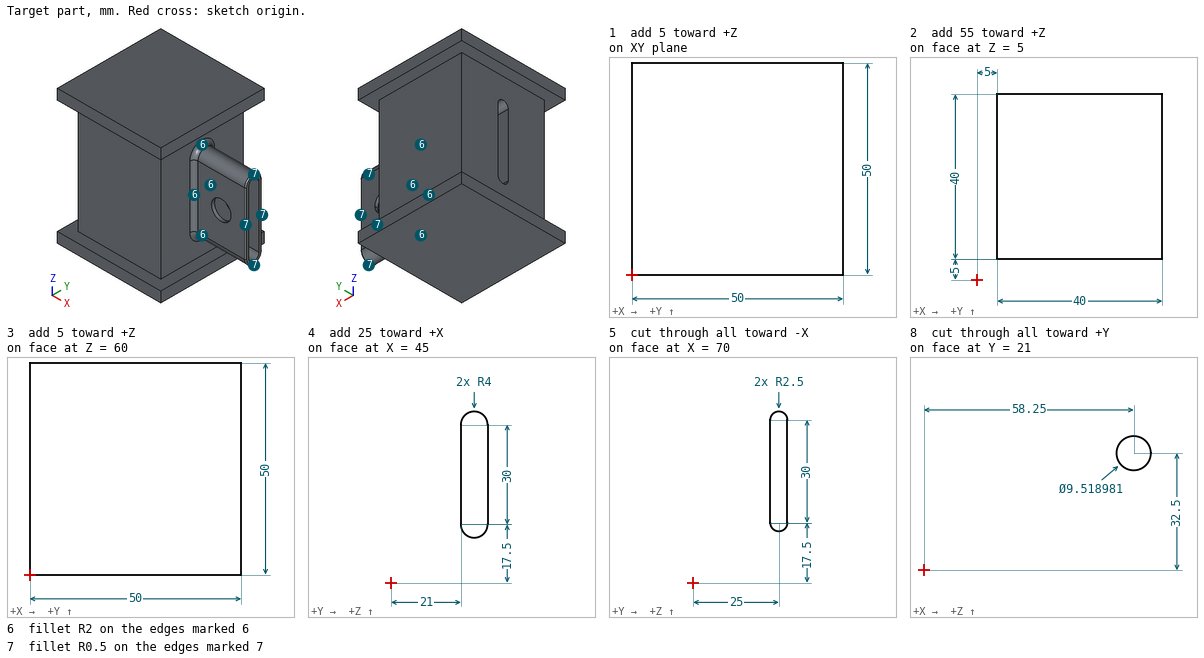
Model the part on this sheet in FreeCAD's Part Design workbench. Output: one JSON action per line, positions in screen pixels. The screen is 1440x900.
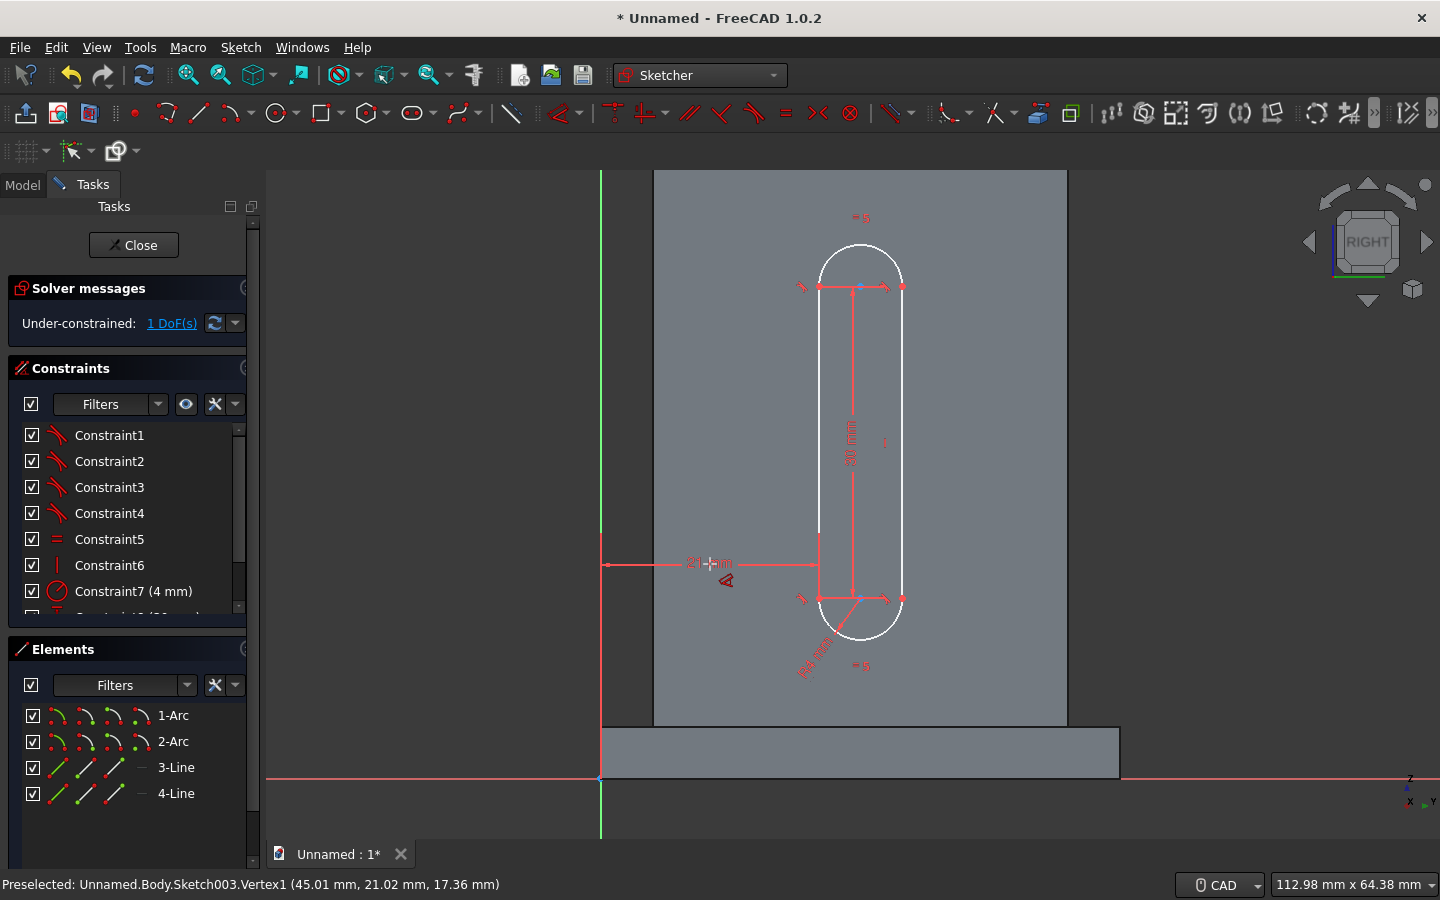
{"action": "left_click", "coordinate": [819, 598]}
{"action": "left_click", "coordinate": [567, 688]}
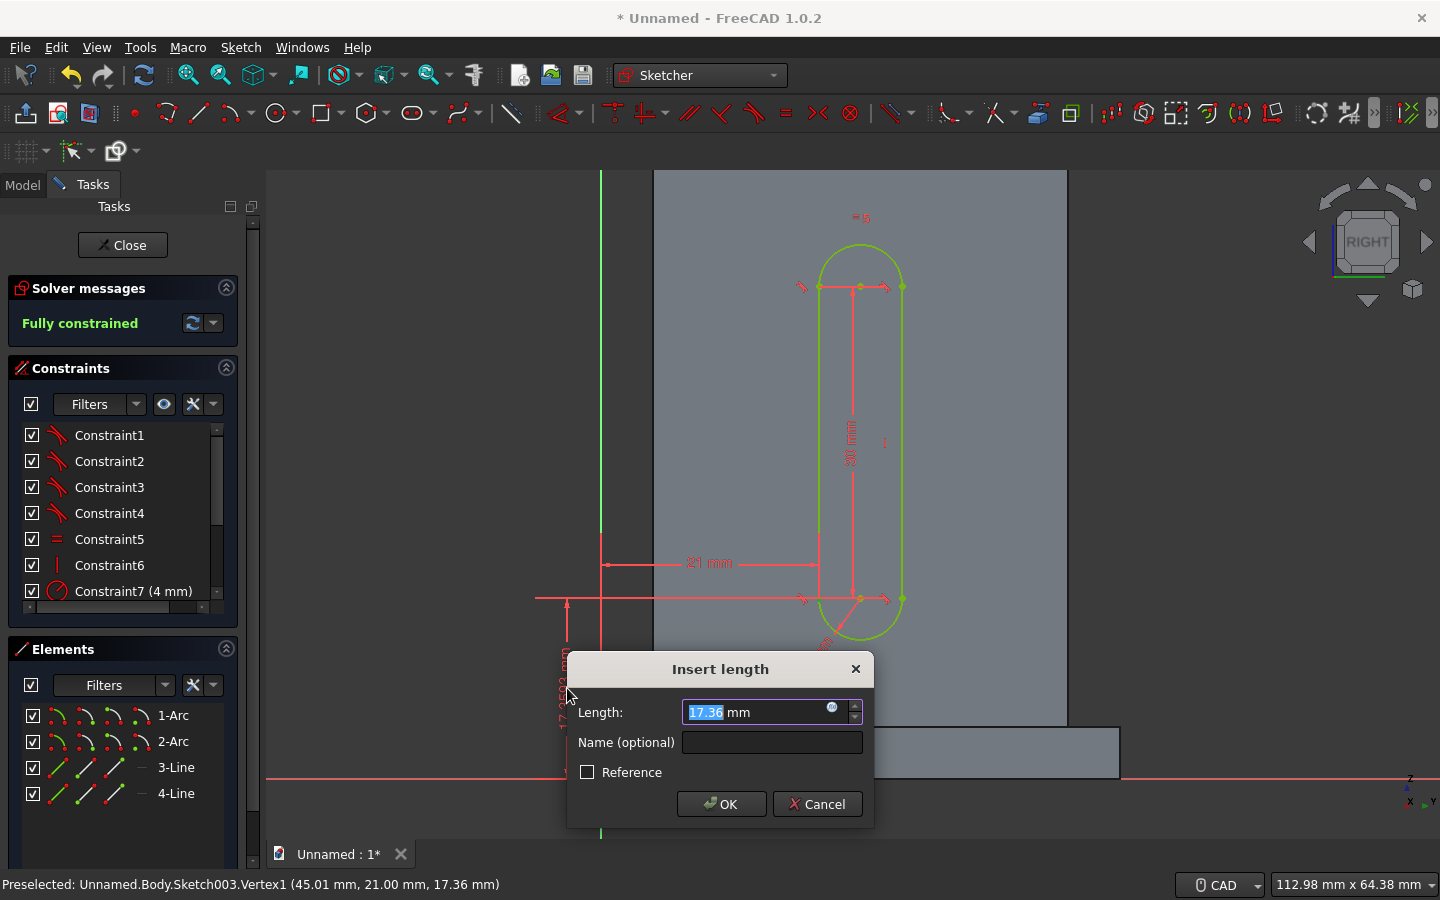
{"action": "type", "text": "17.5"}
{"action": "key", "text": "Return"}
{"action": "key", "text": "Escape"}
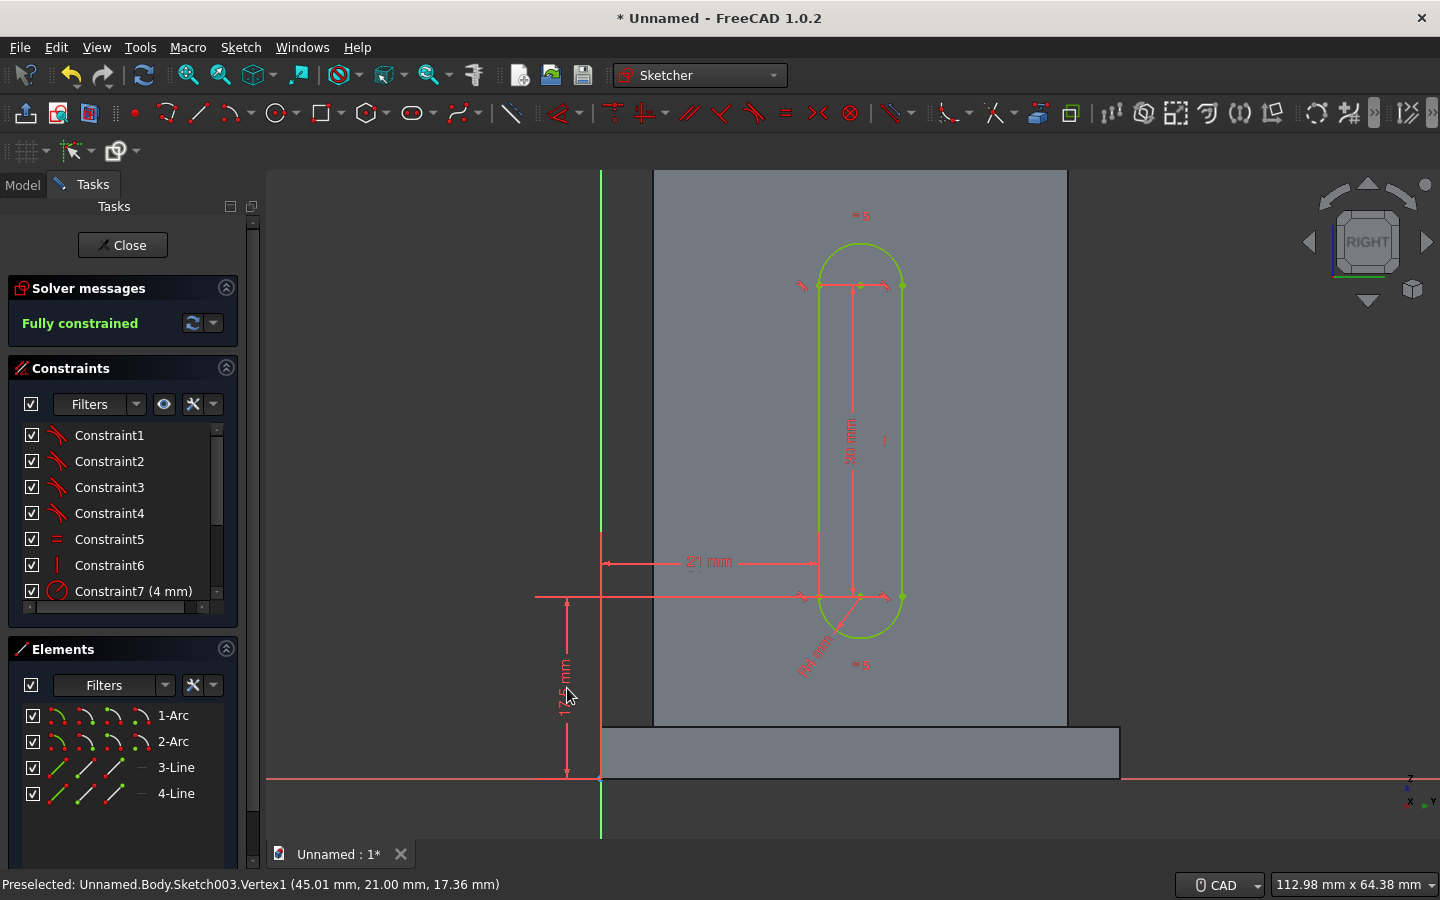
{"action": "left_click", "coordinate": [123, 245]}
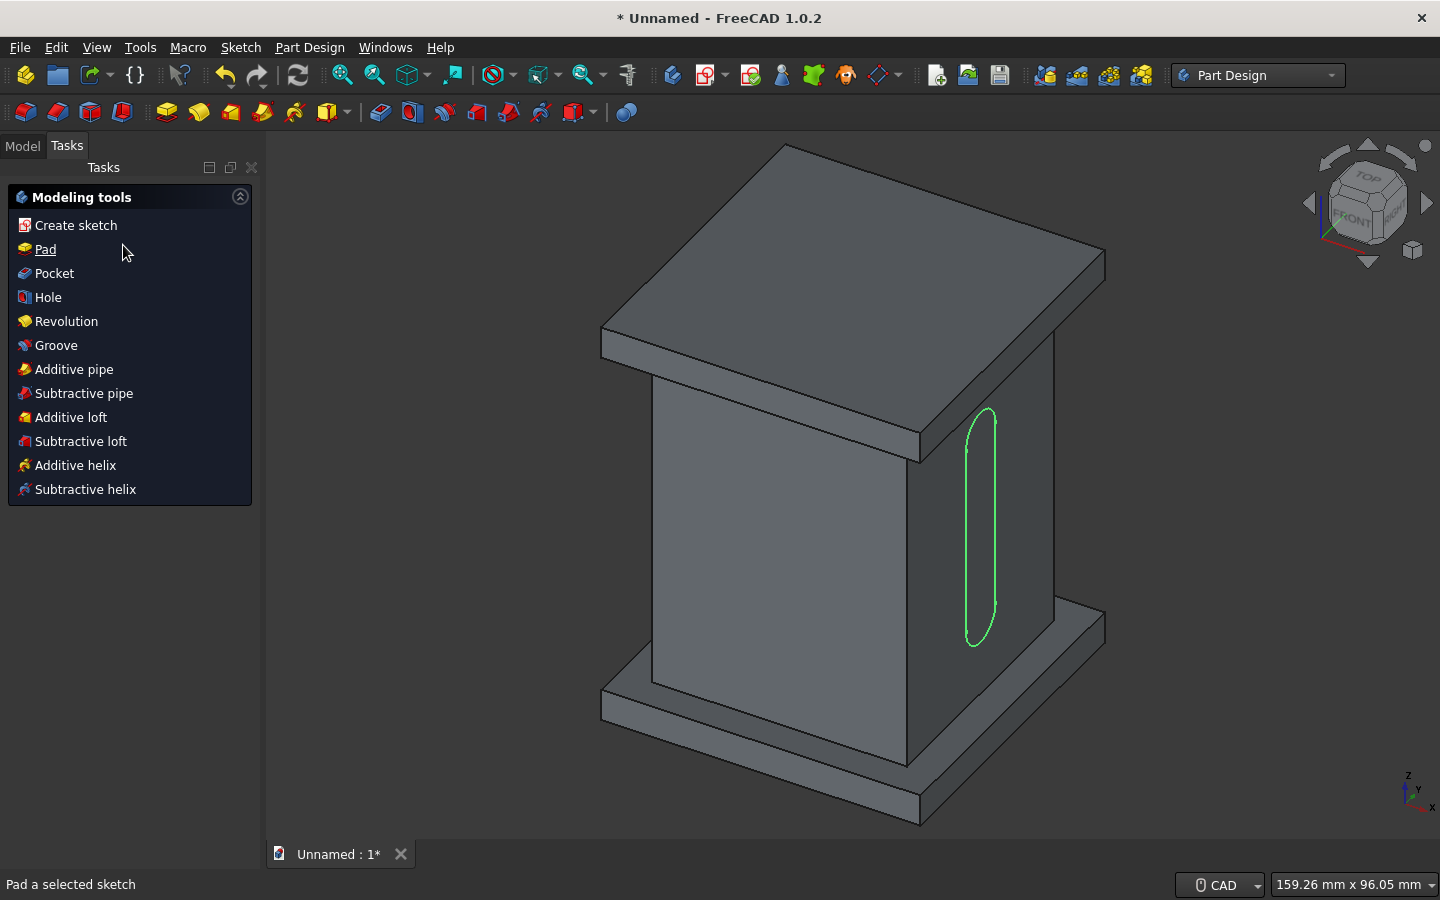
{"action": "left_click", "coordinate": [168, 112]}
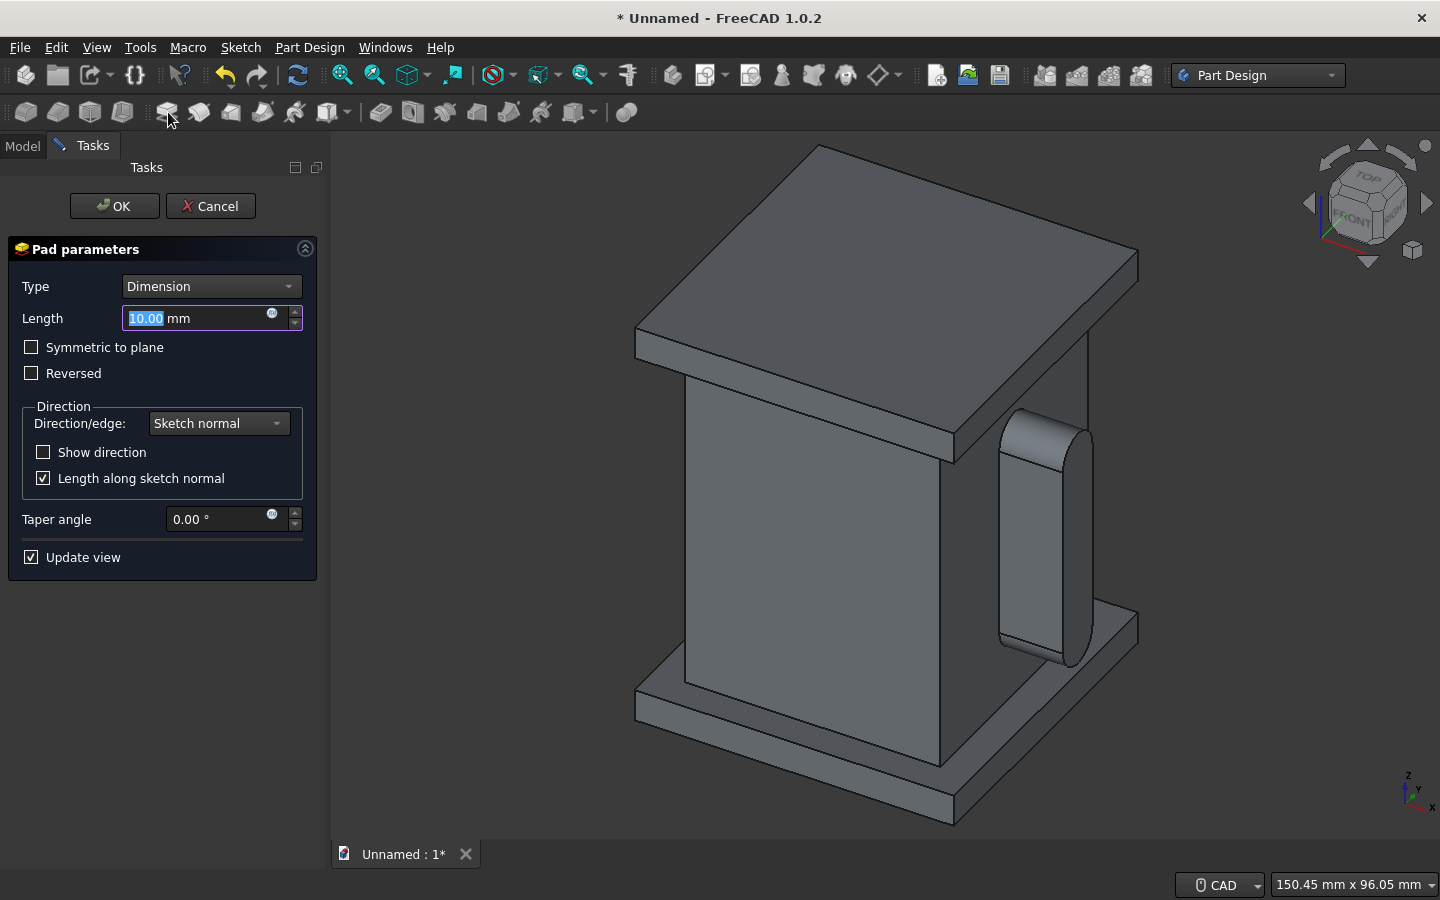
{"action": "type", "text": "25"}
{"action": "key", "text": "Tab"}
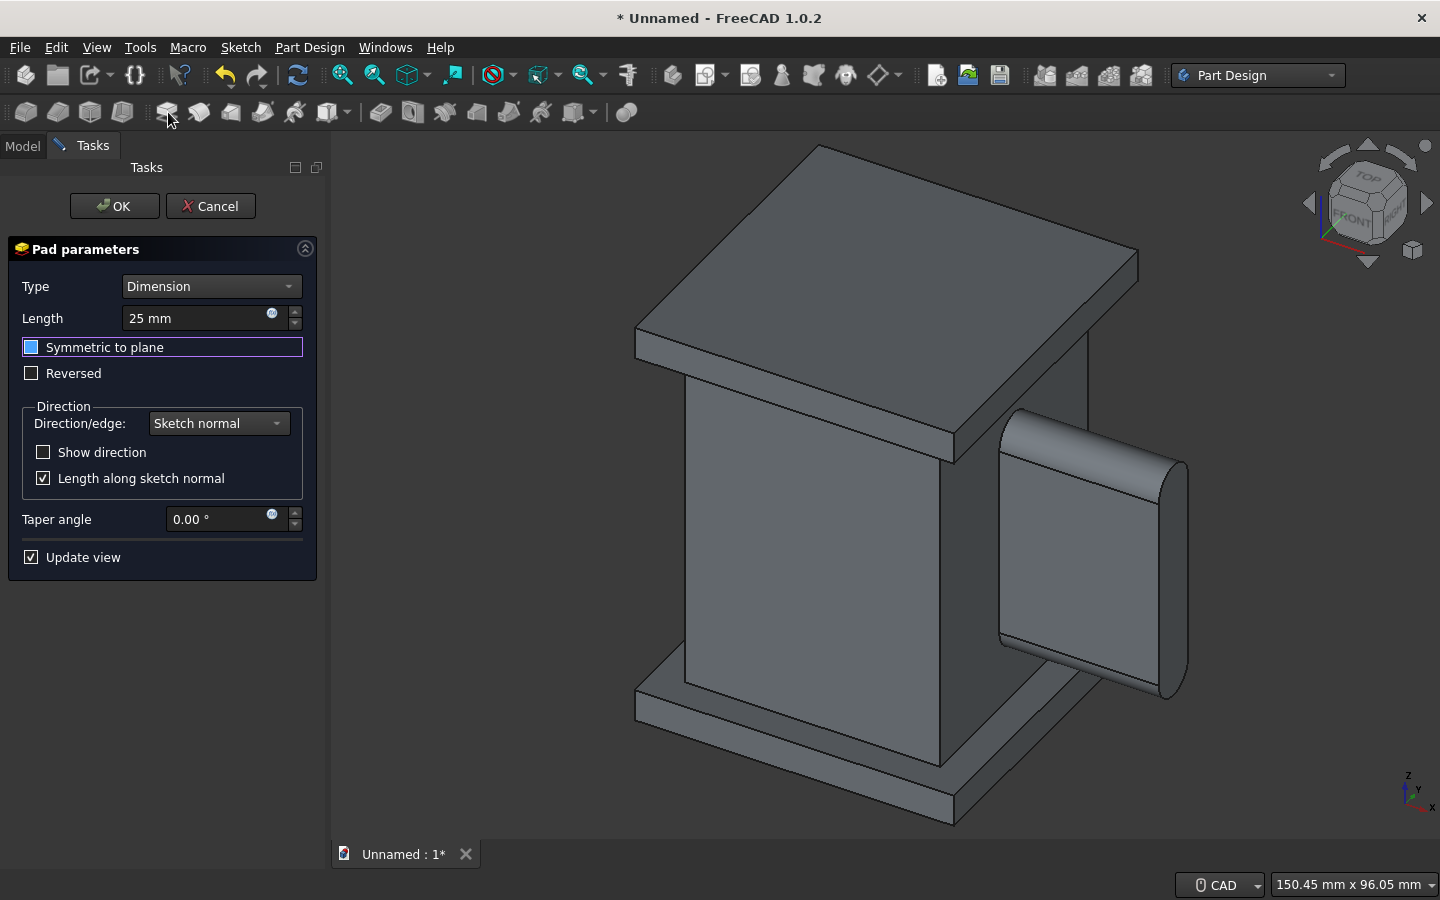
{"action": "left_click", "coordinate": [115, 206]}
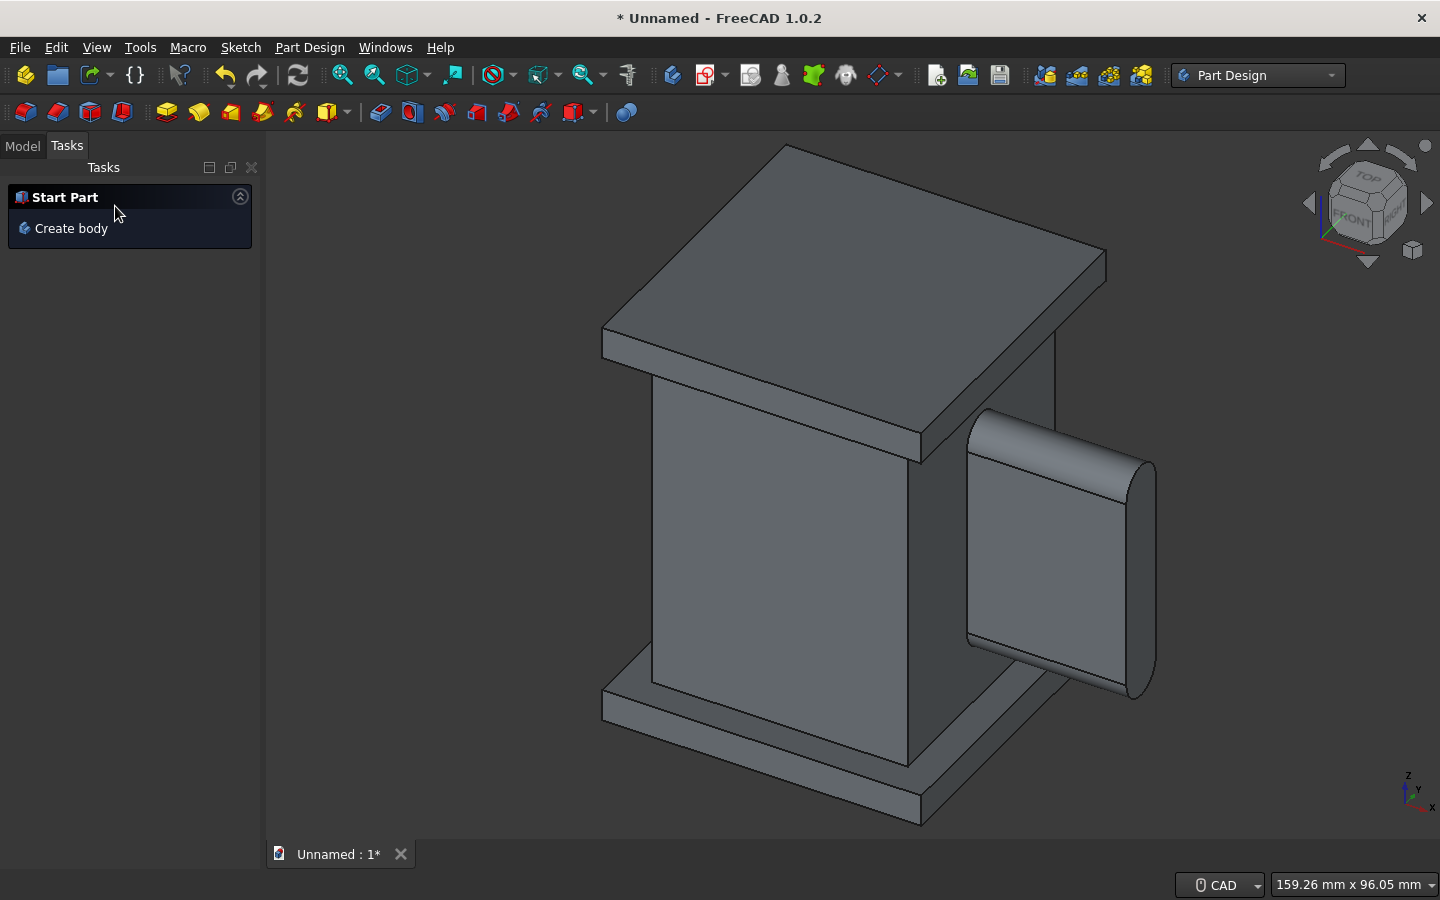
{"action": "left_click", "coordinate": [344, 76]}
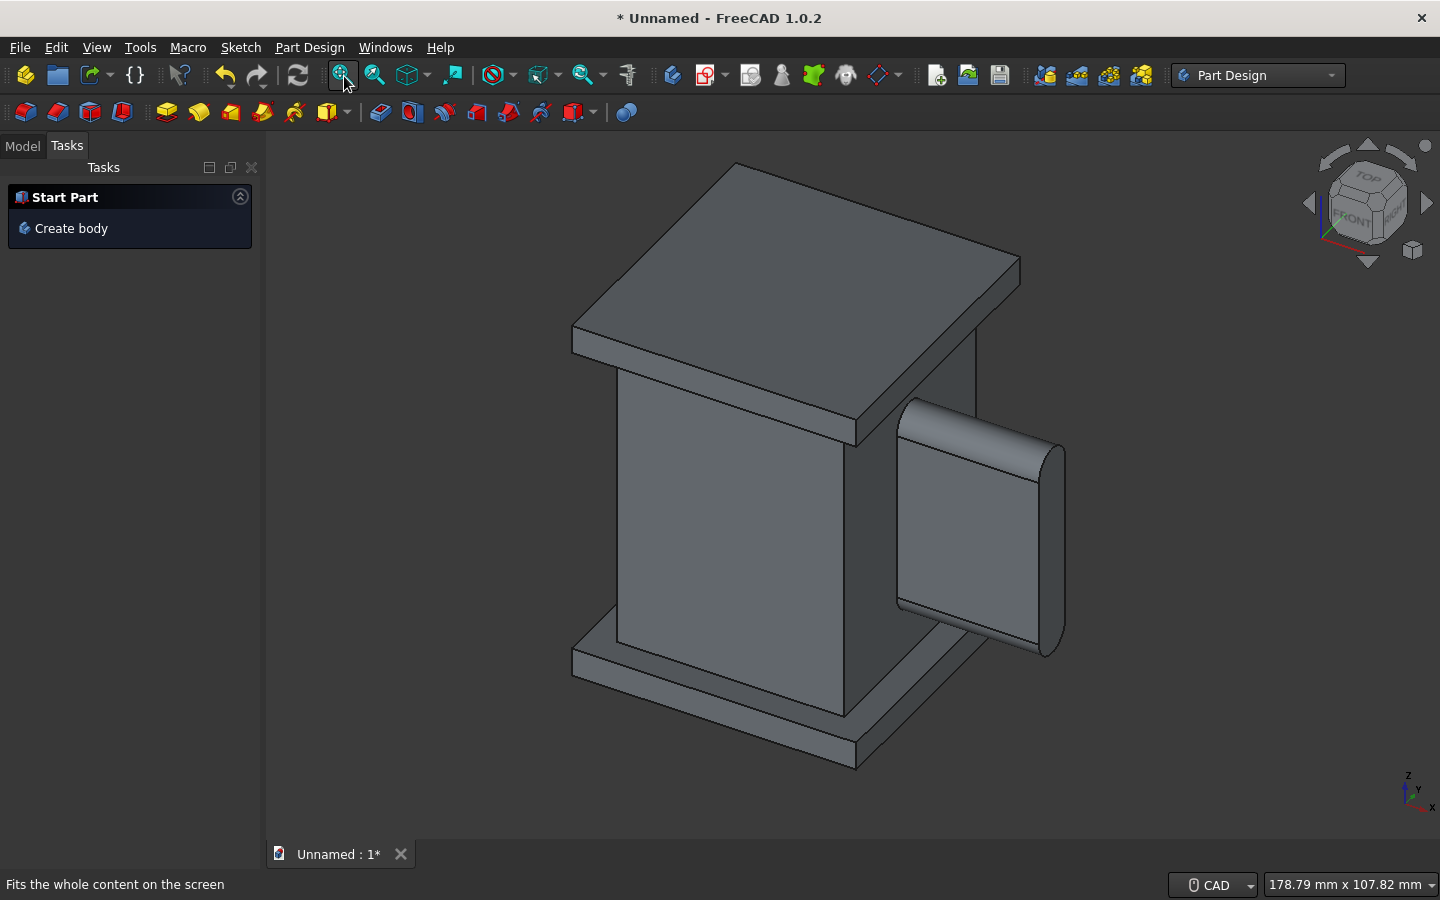
{"action": "left_click", "coordinate": [1052, 608]}